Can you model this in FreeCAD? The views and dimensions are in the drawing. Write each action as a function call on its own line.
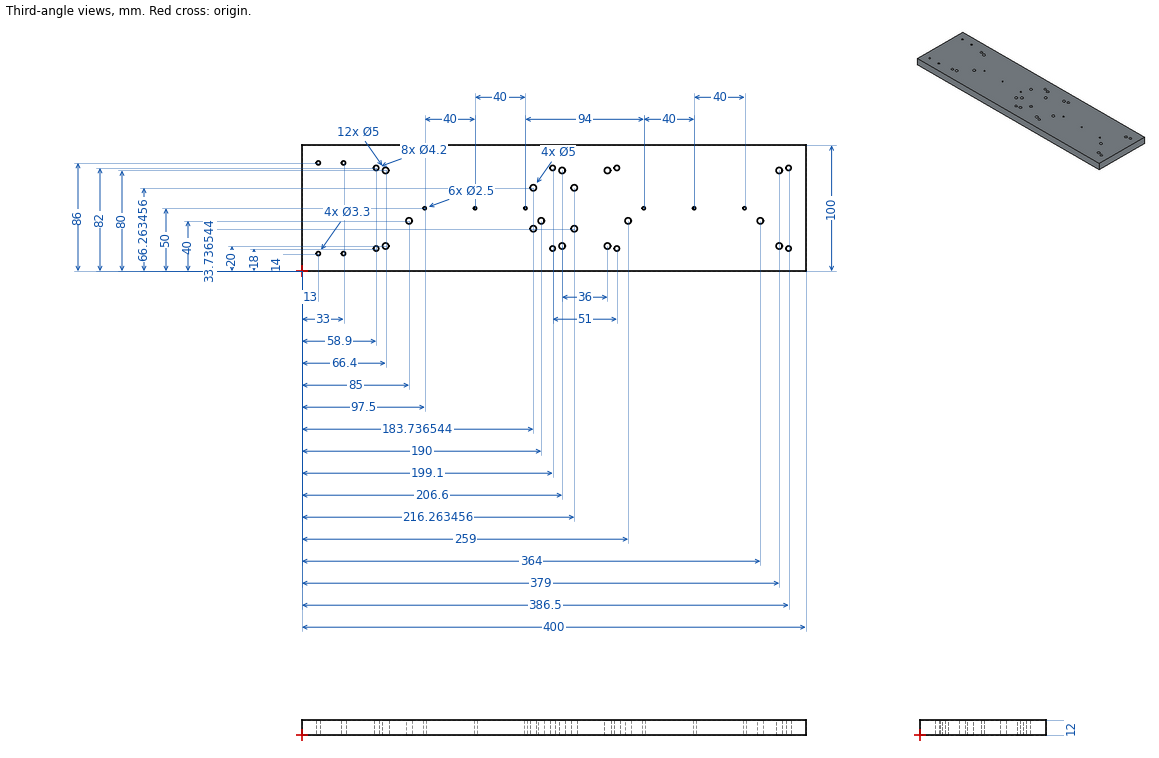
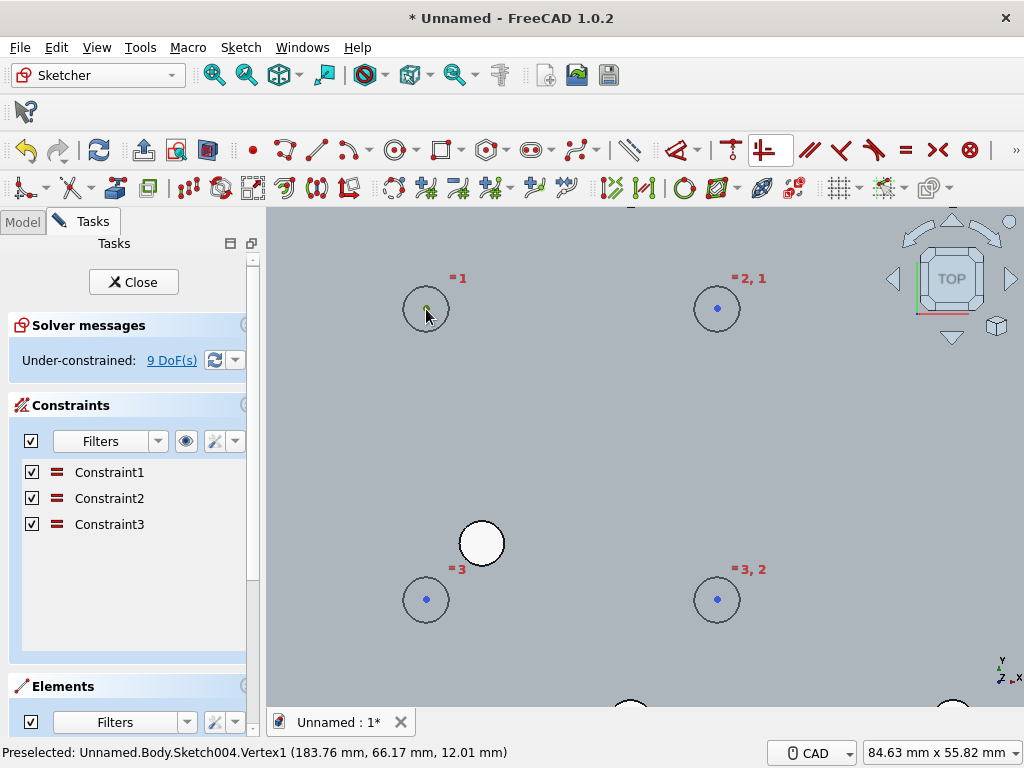
click(717, 309)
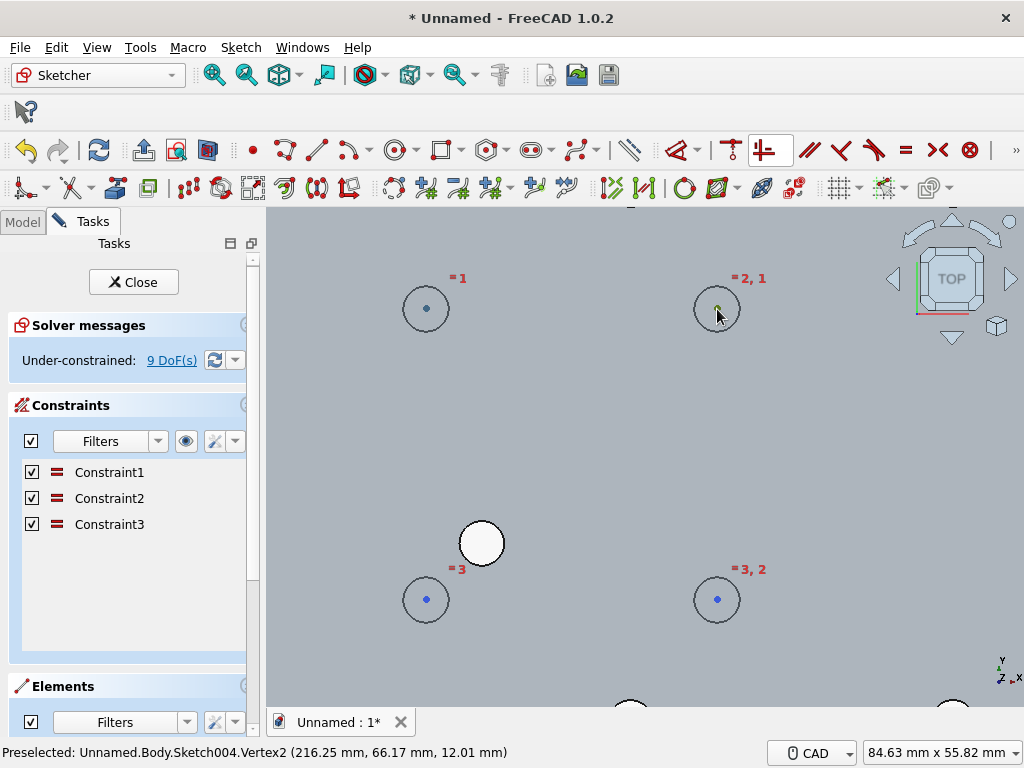
click(788, 150)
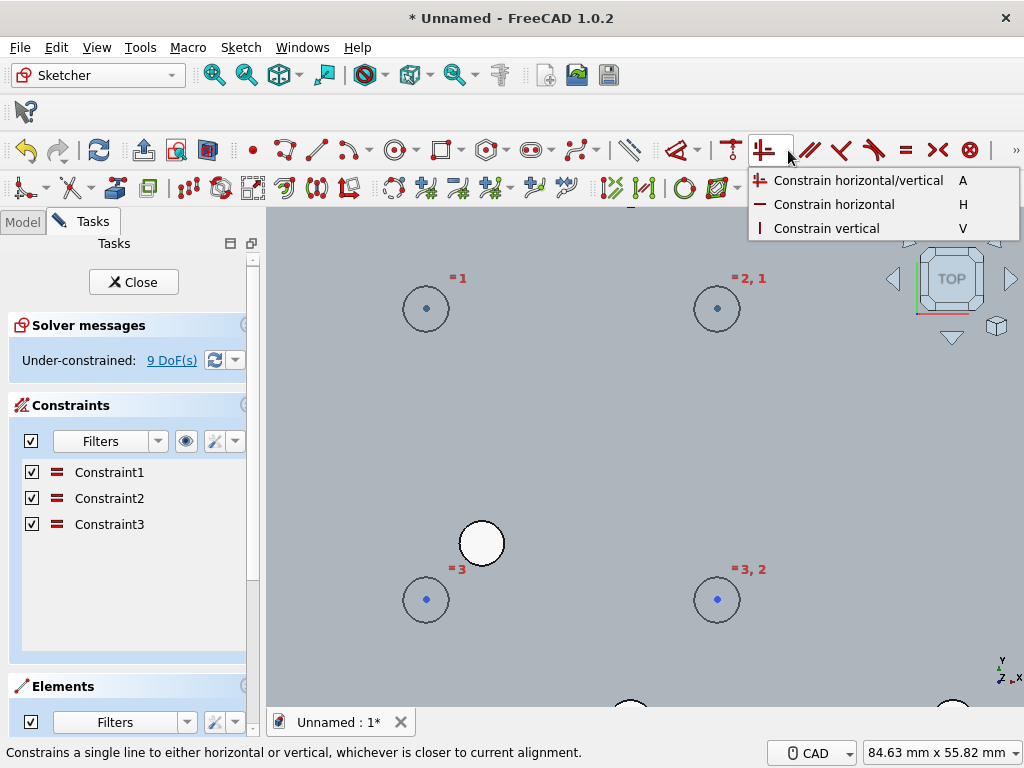
click(884, 204)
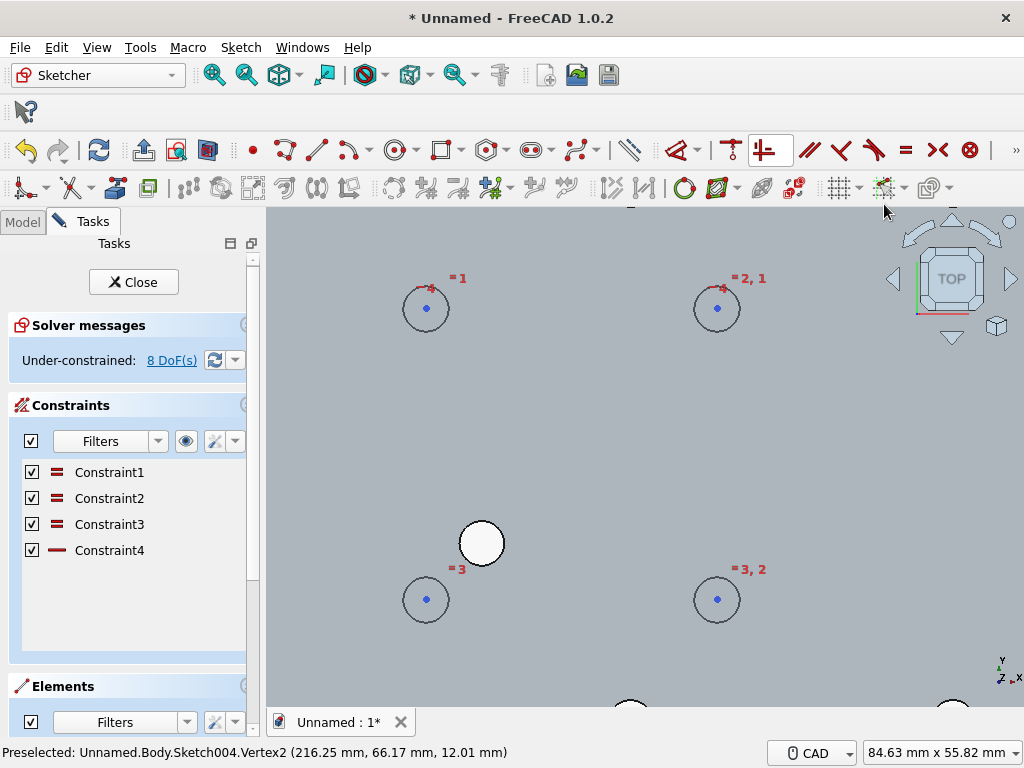
click(717, 309)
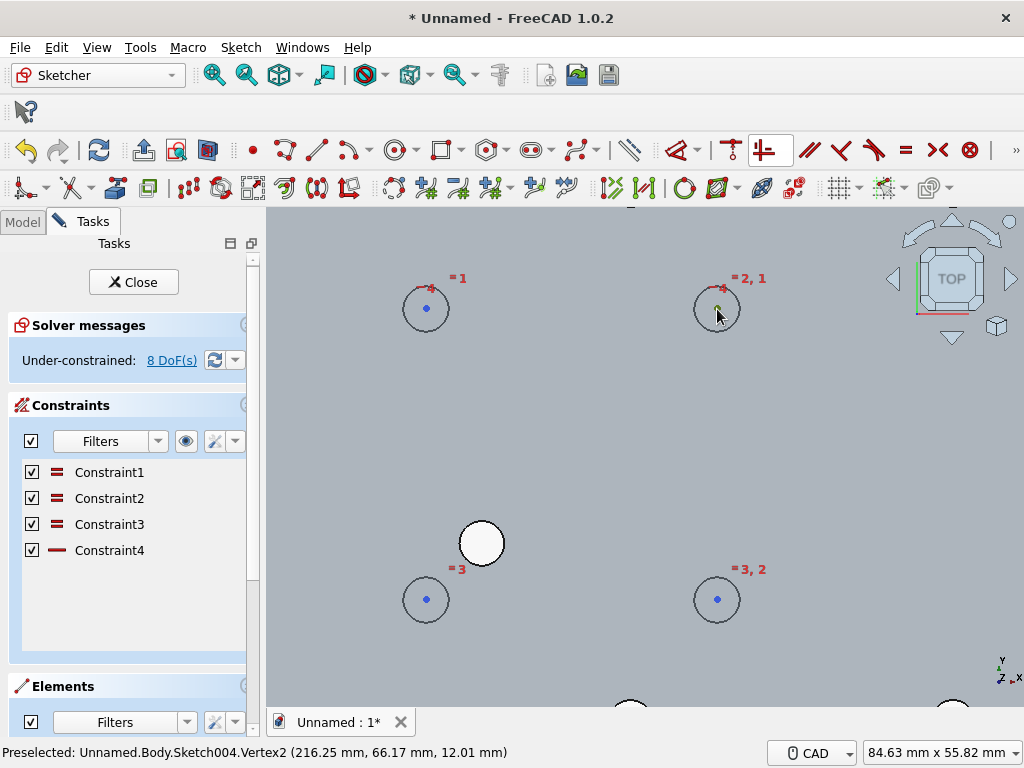
click(717, 600)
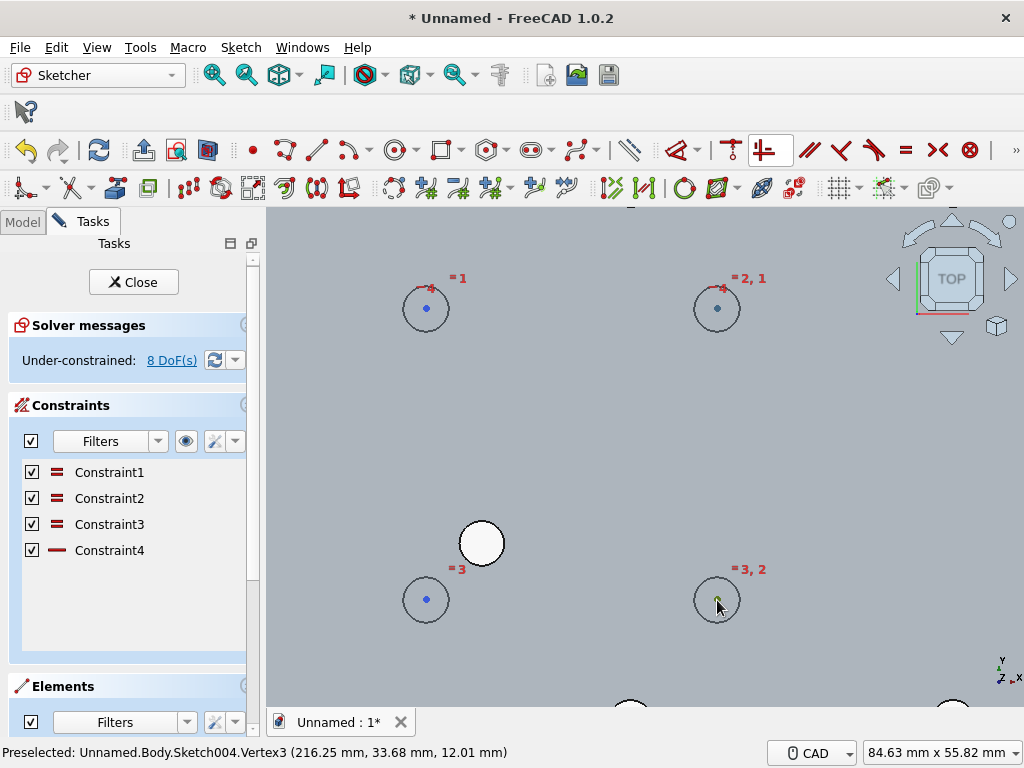
key(v)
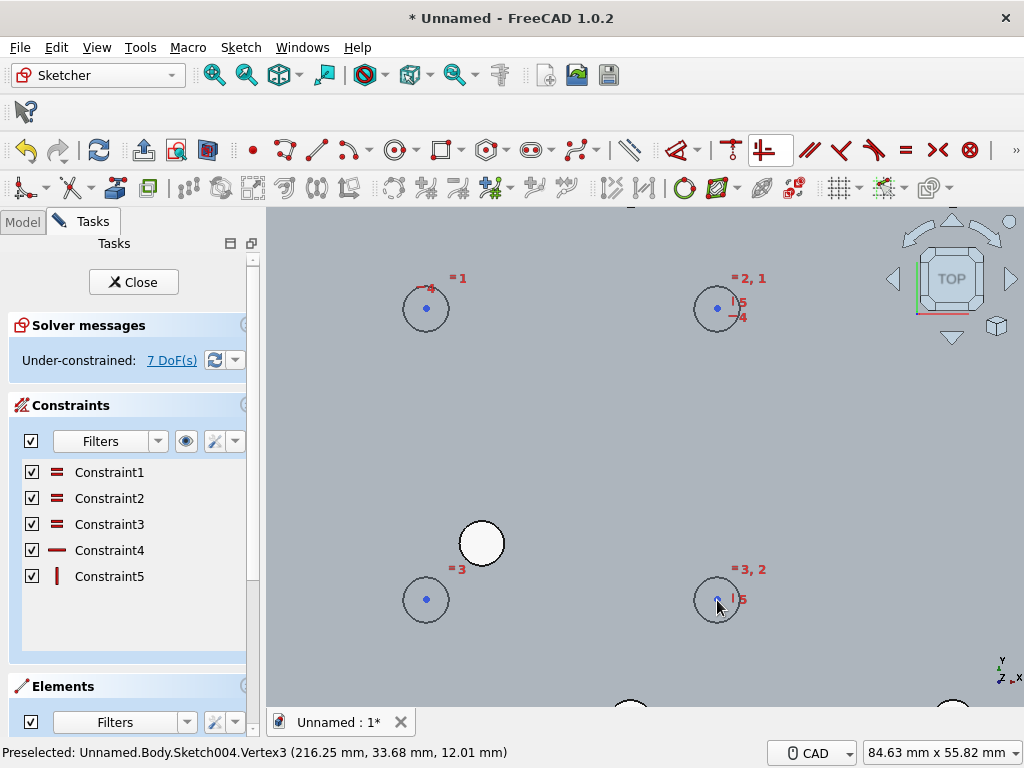
click(426, 309)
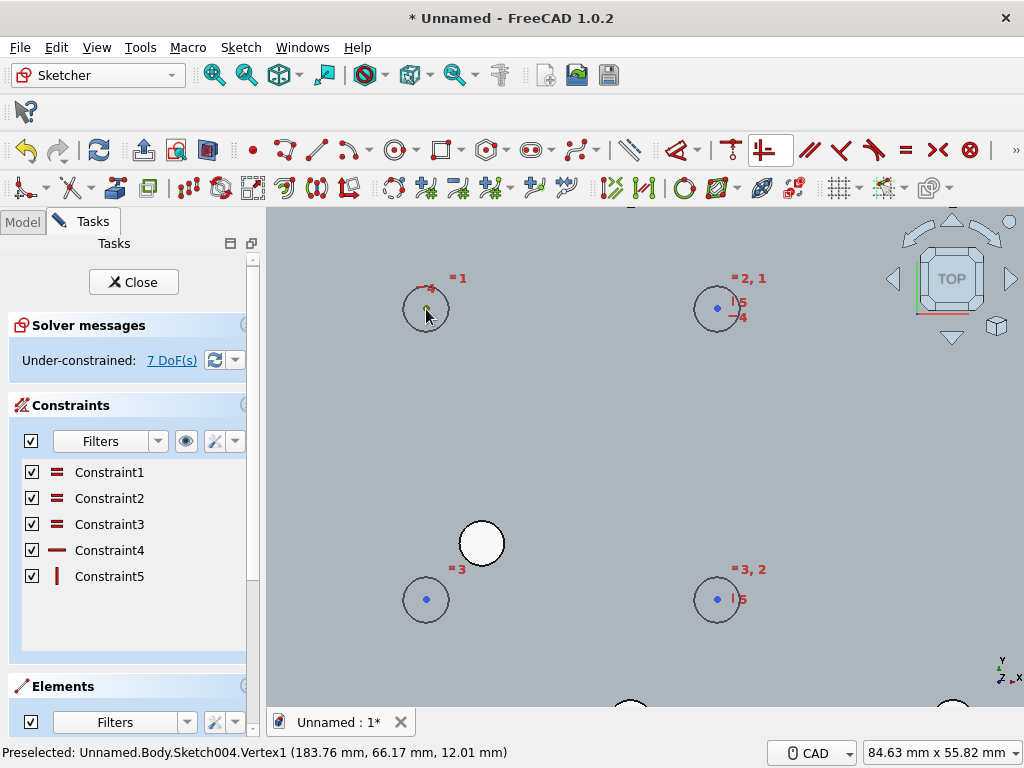
click(426, 600)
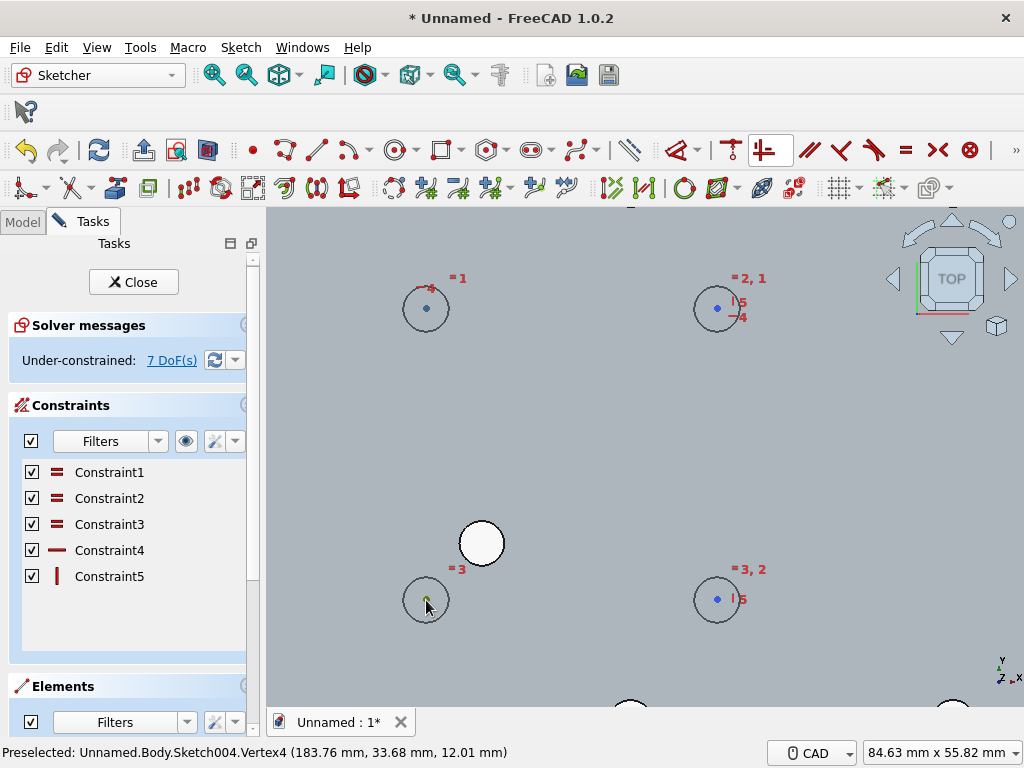
click(788, 150)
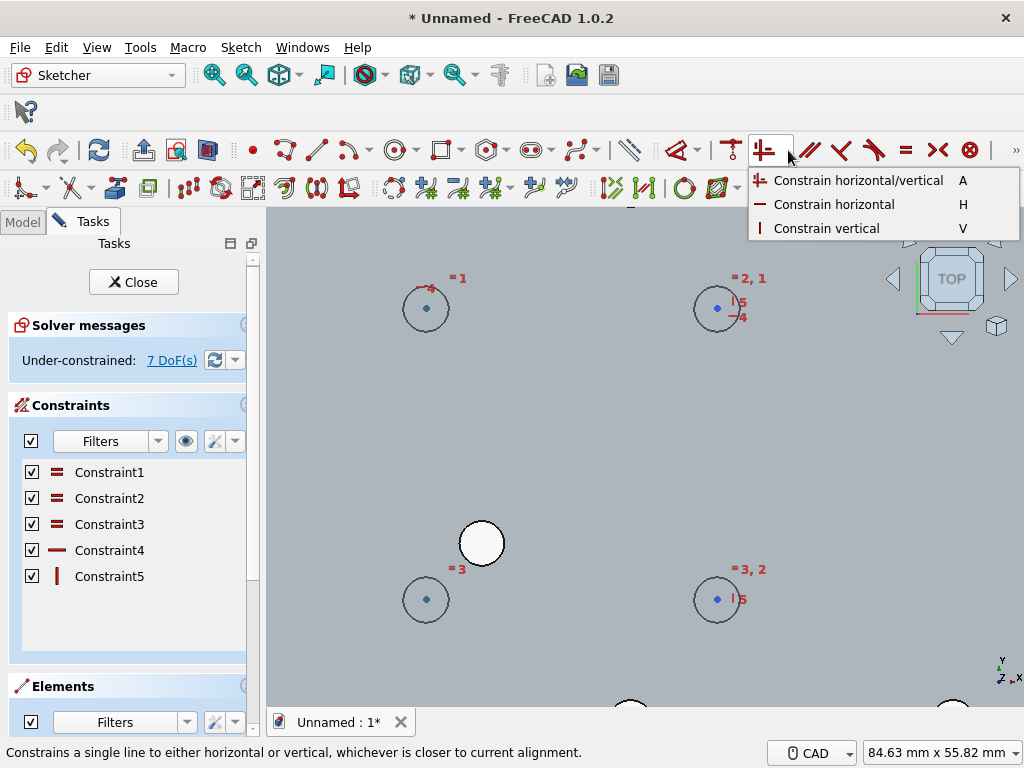
click(884, 228)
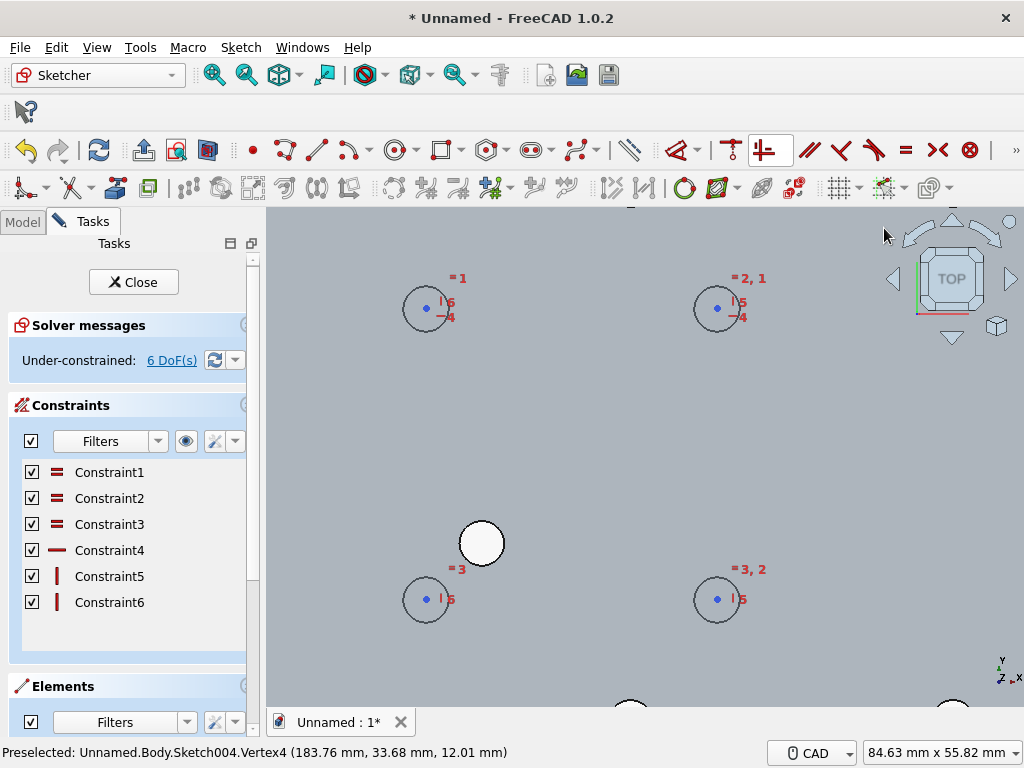
click(717, 600)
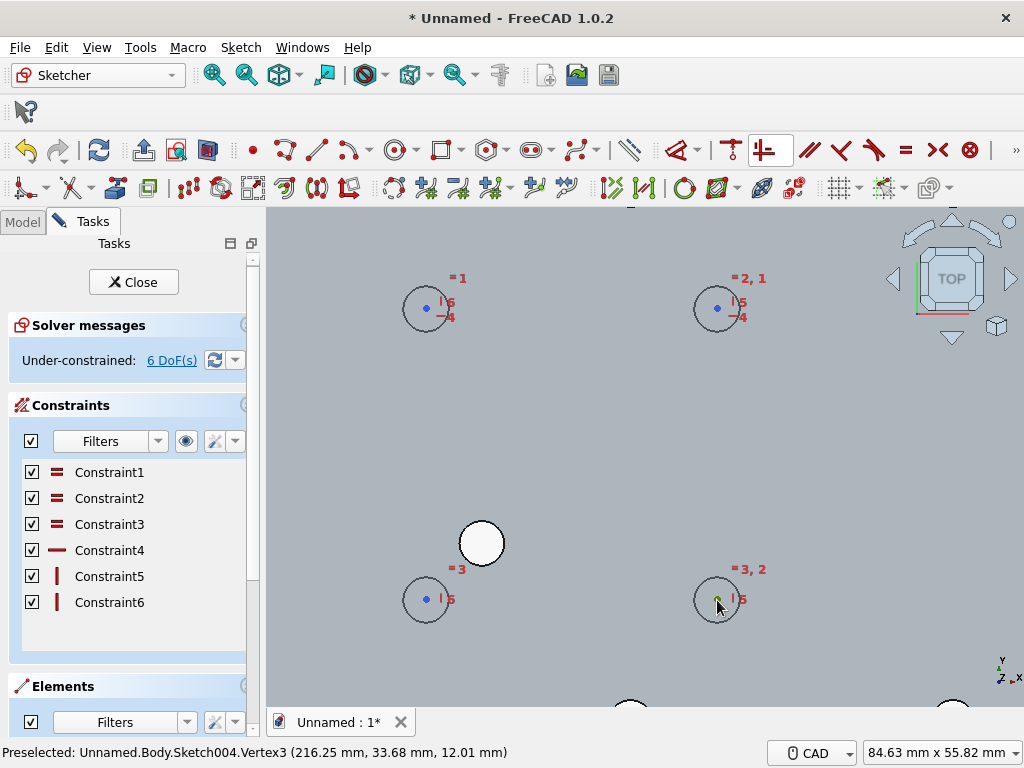
click(426, 600)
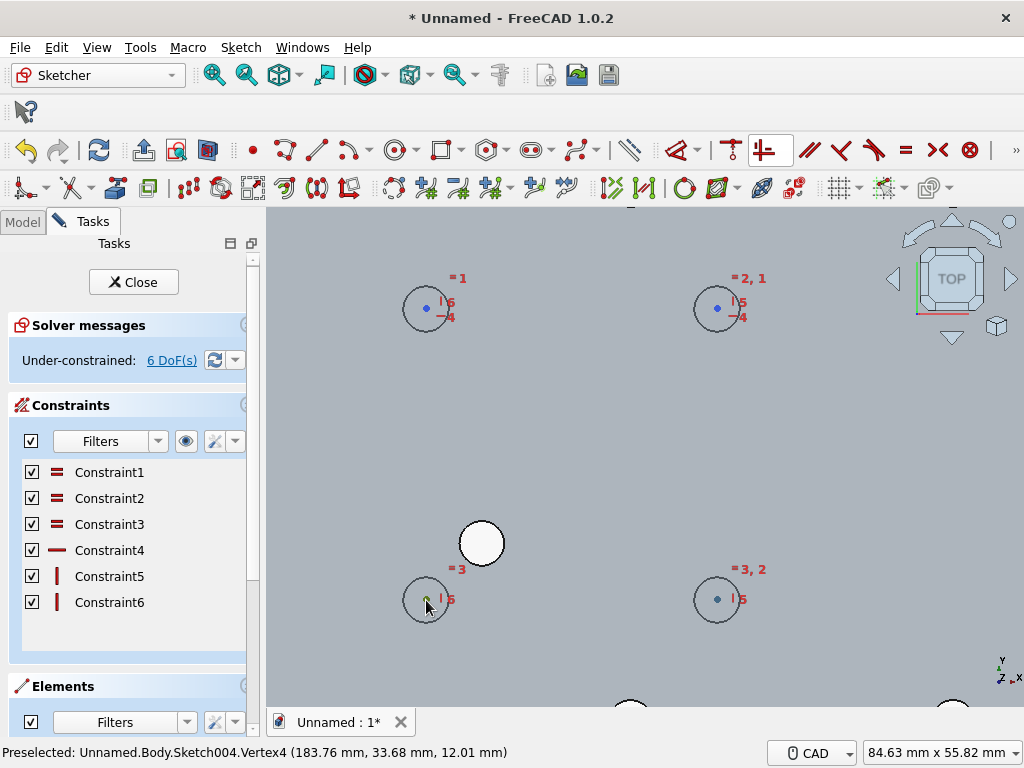
click(788, 150)